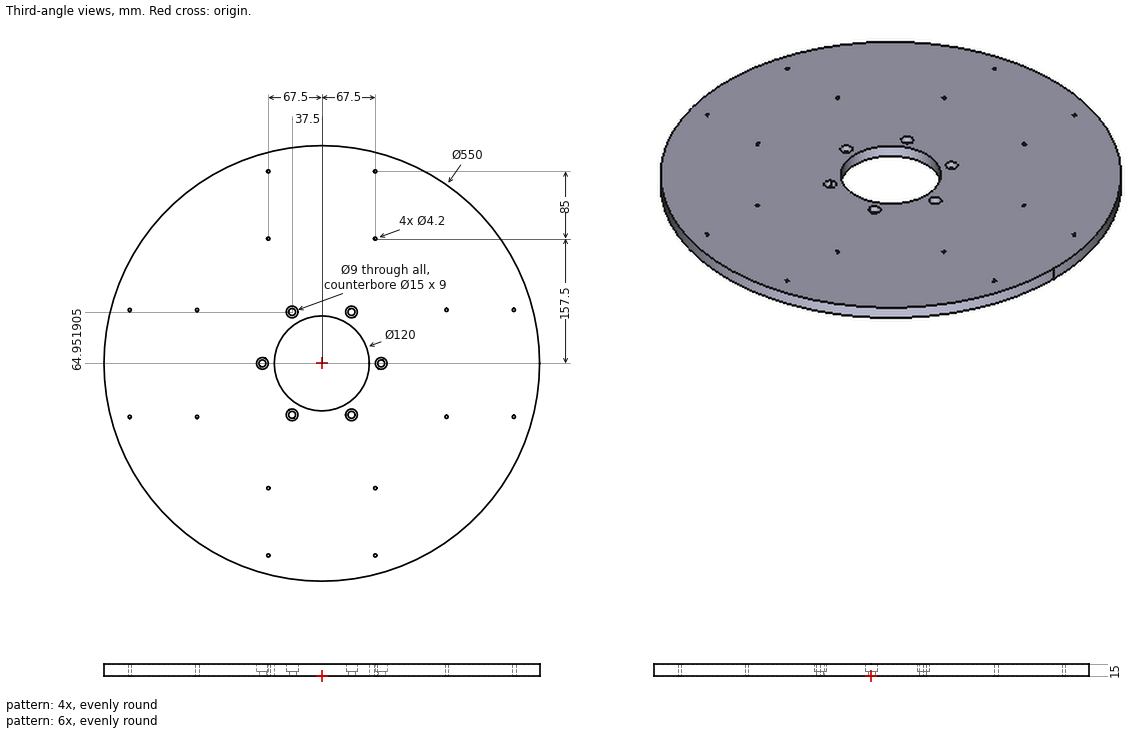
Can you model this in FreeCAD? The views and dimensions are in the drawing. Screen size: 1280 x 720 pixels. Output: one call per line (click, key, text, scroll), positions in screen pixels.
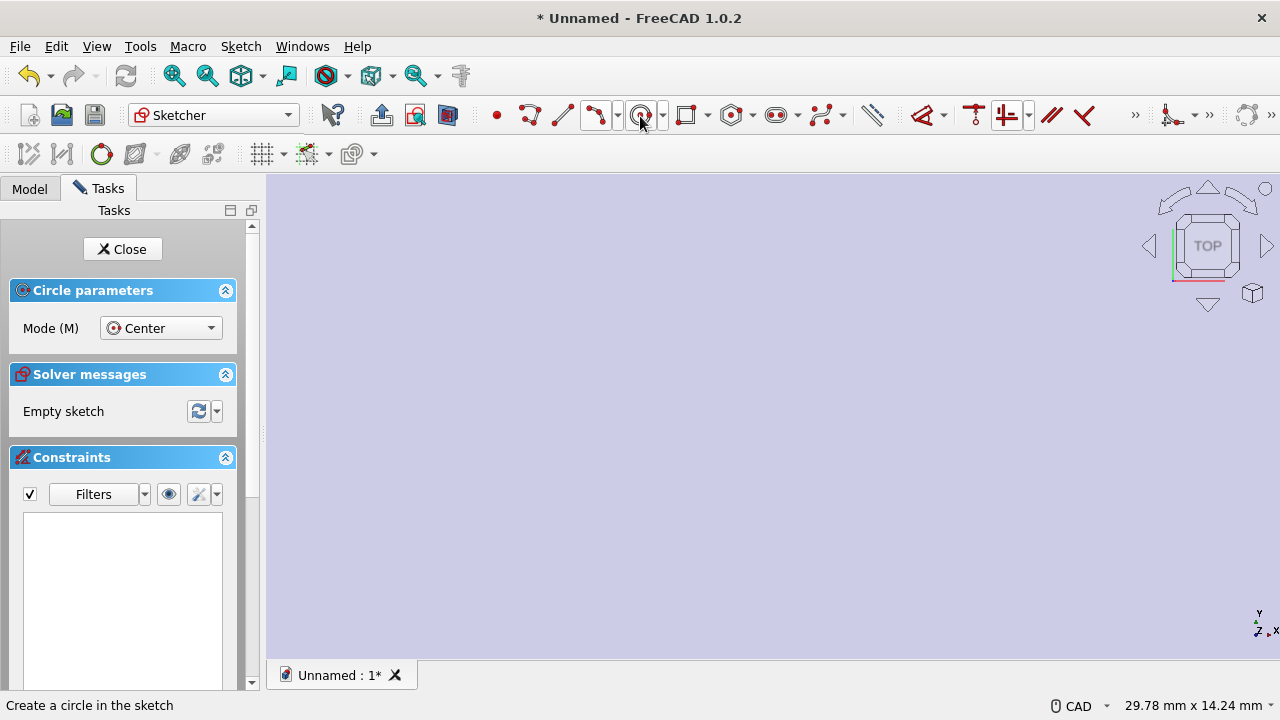
click(703, 416)
move(811, 307)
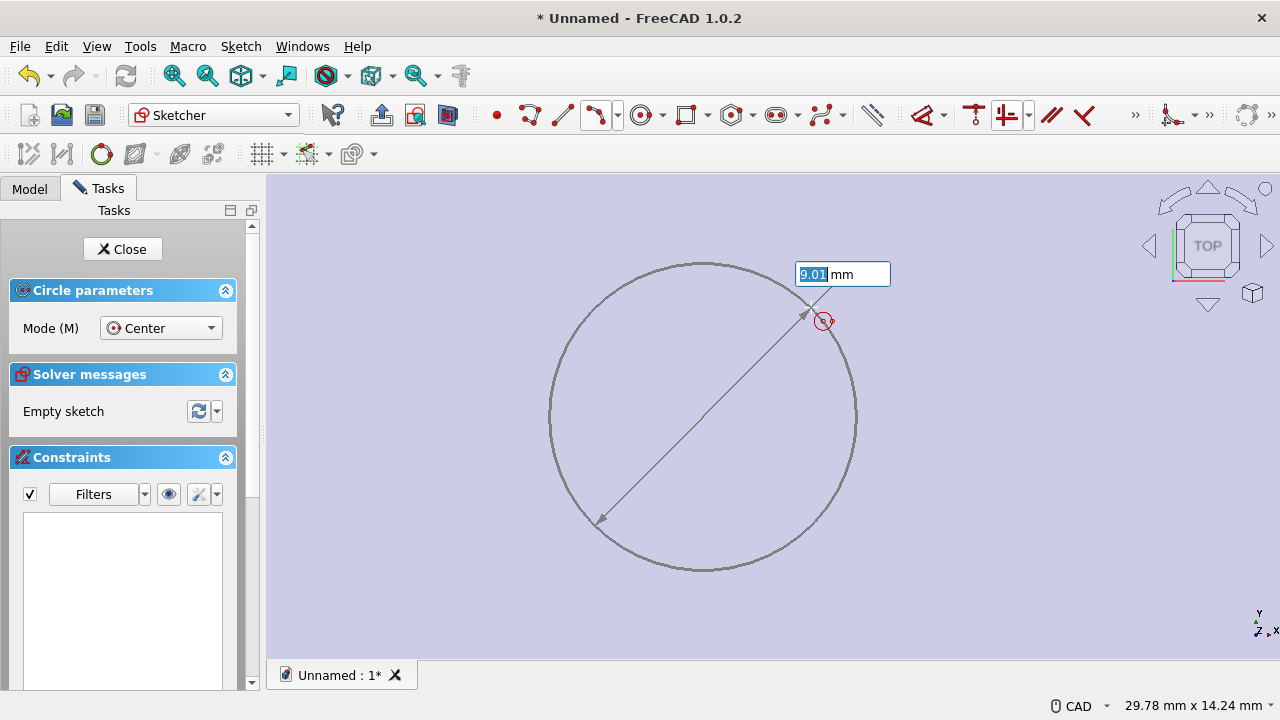
text(9)
key(Return)
key(Escape)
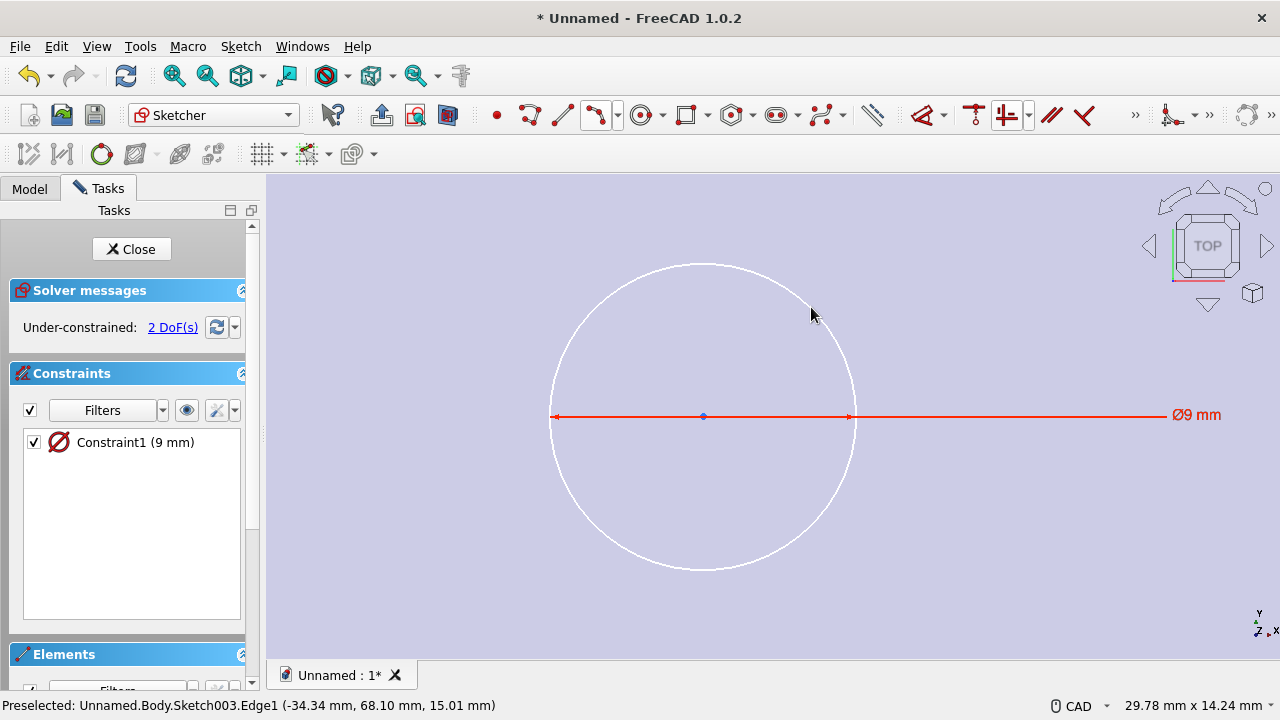
click(922, 116)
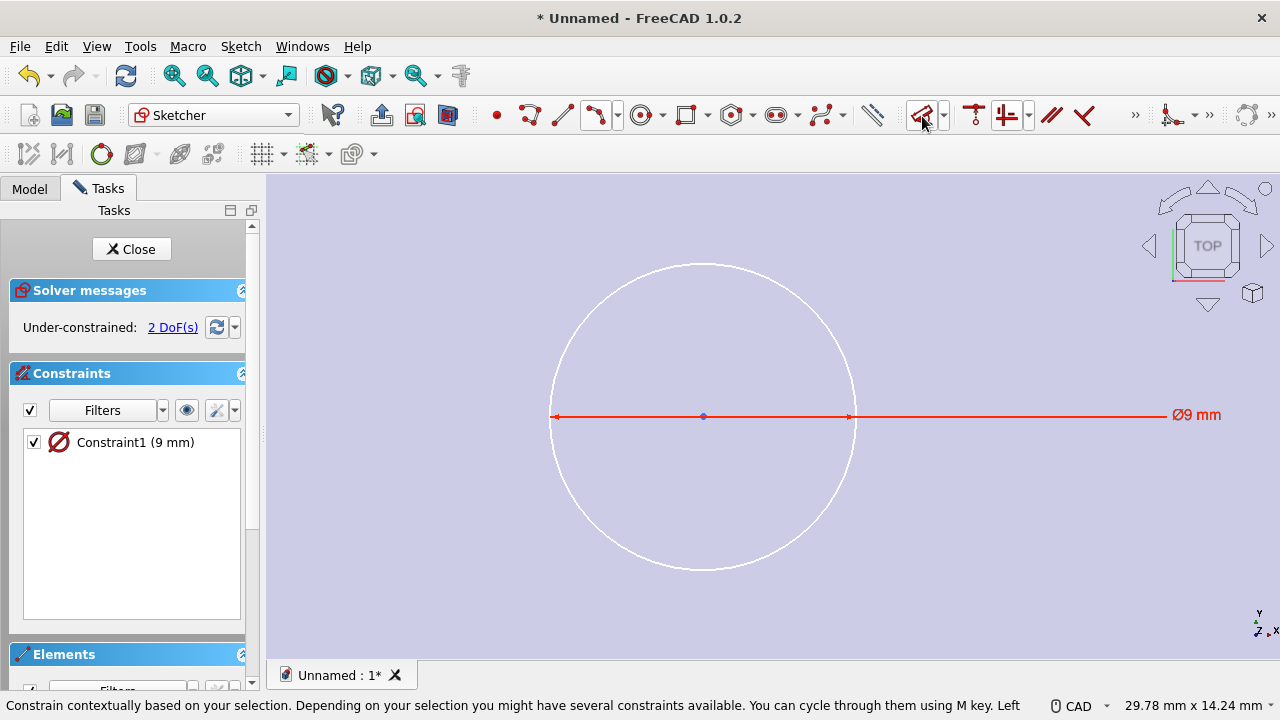
click(703, 417)
click(909, 383)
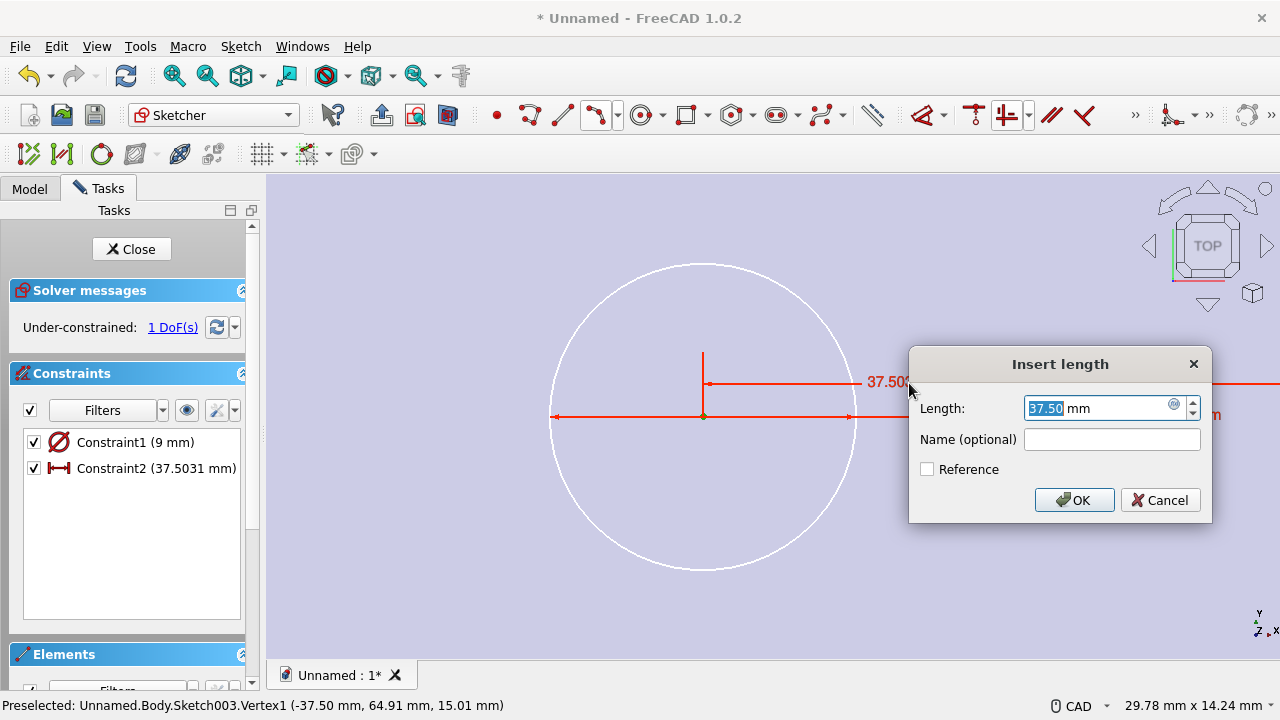
text(37.5)
key(Return)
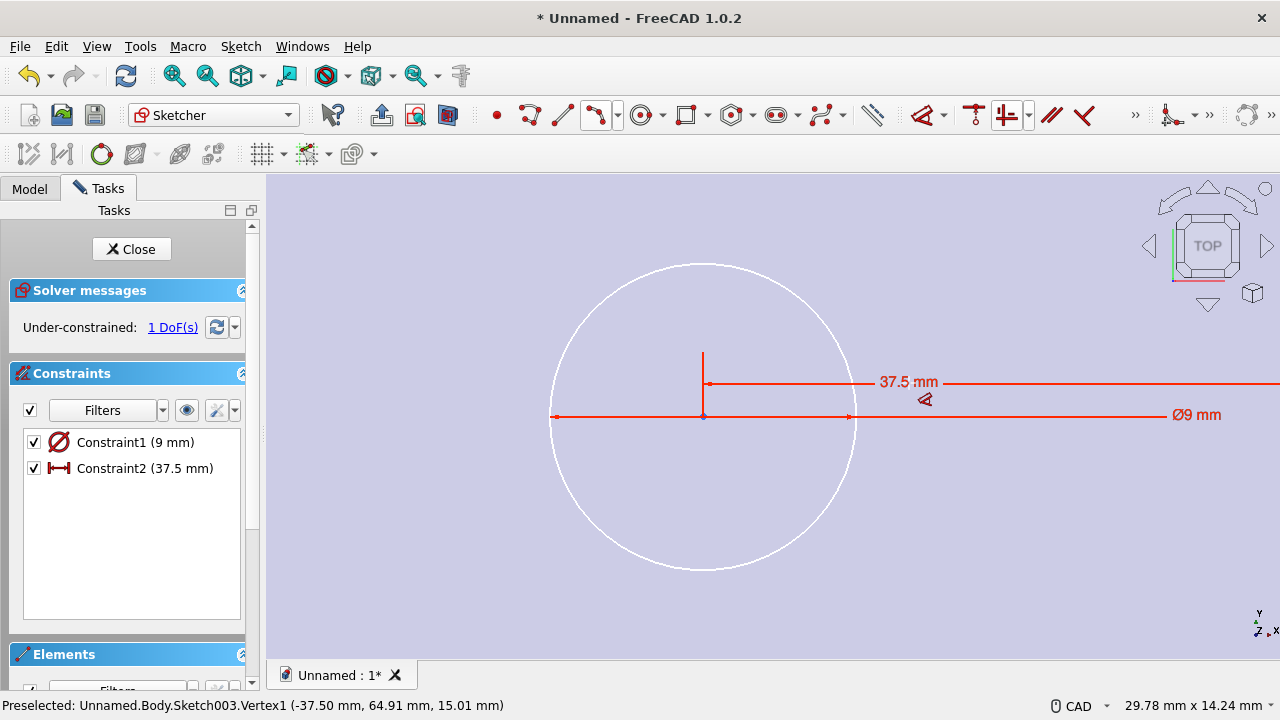
click(703, 417)
click(669, 524)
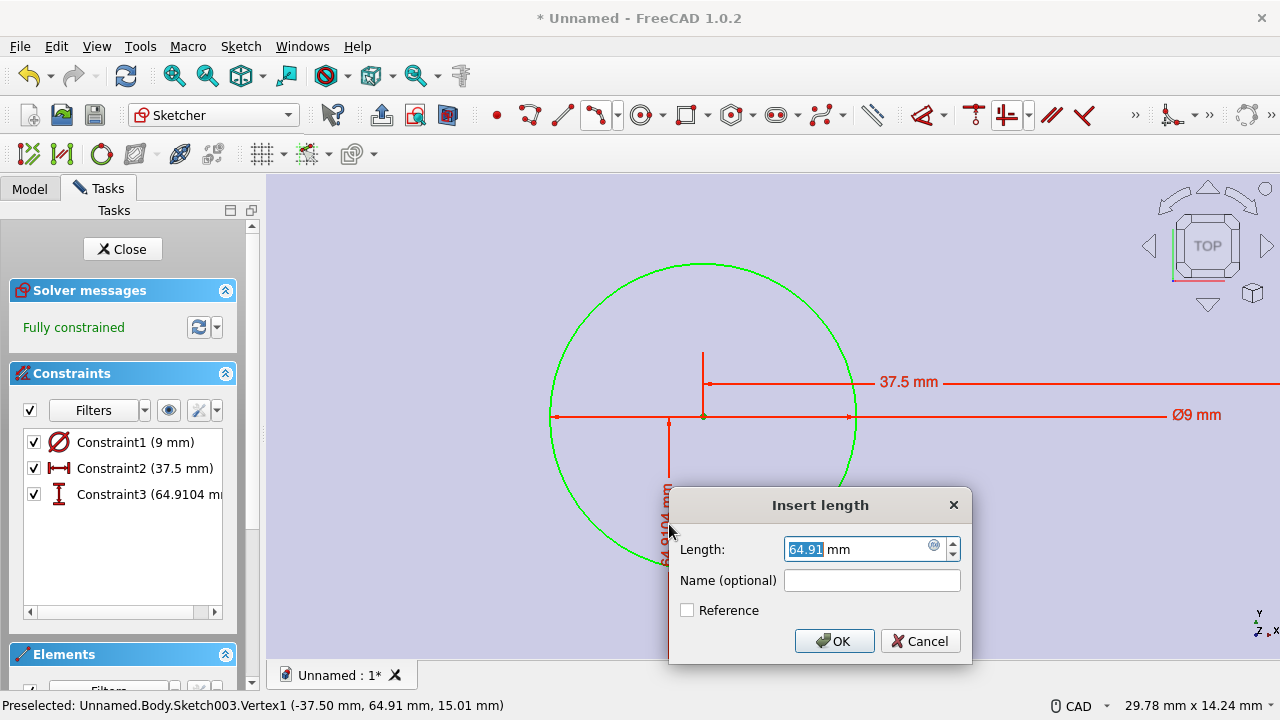
text(64.951905)
key(Return)
key(Escape)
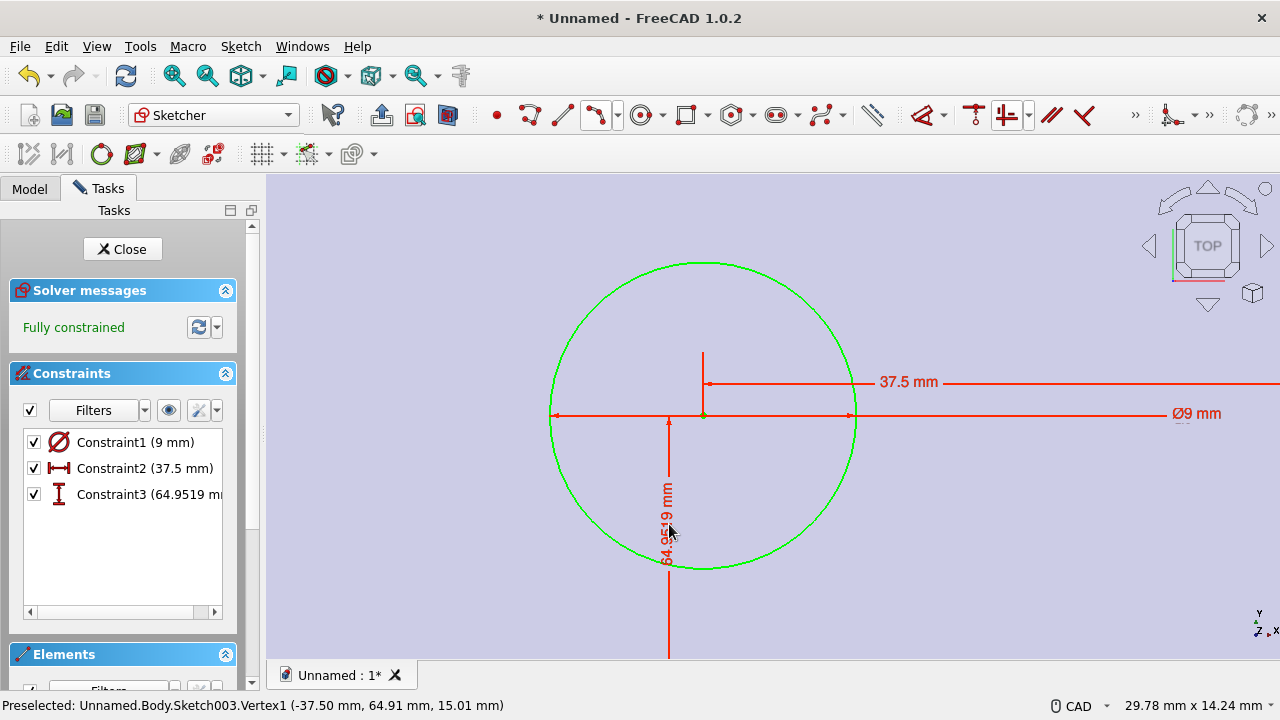
click(123, 249)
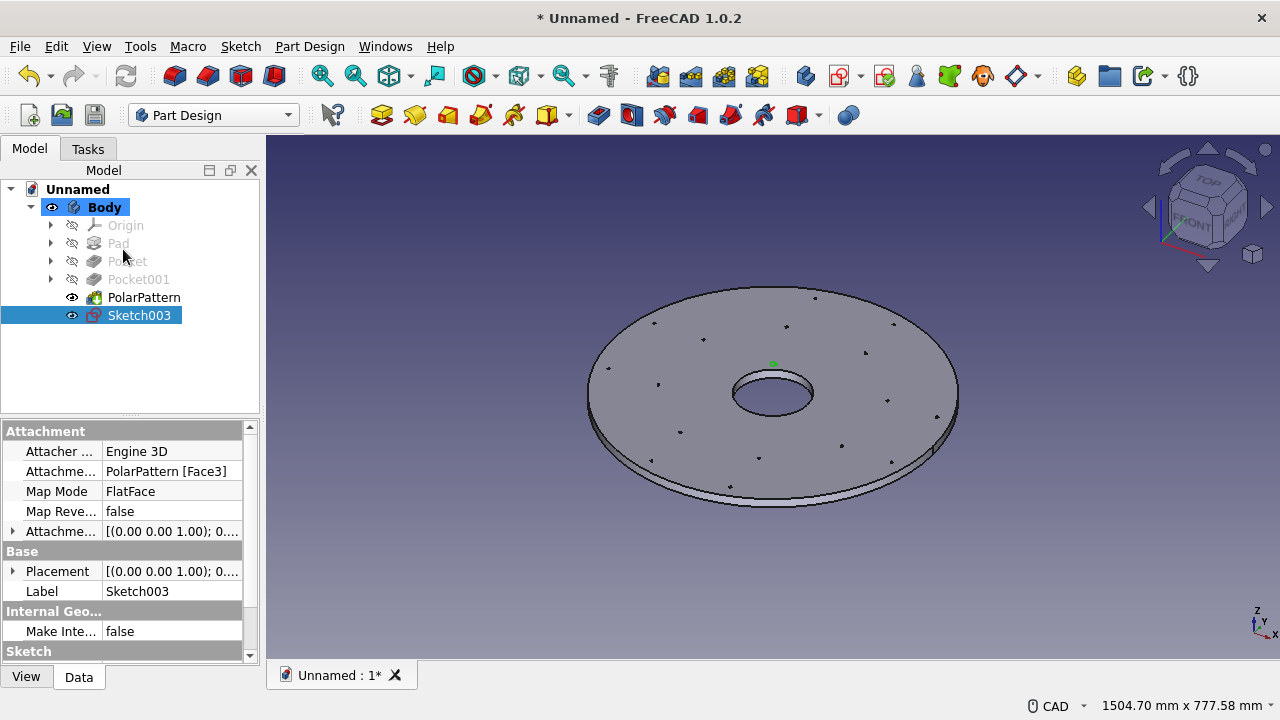
click(632, 116)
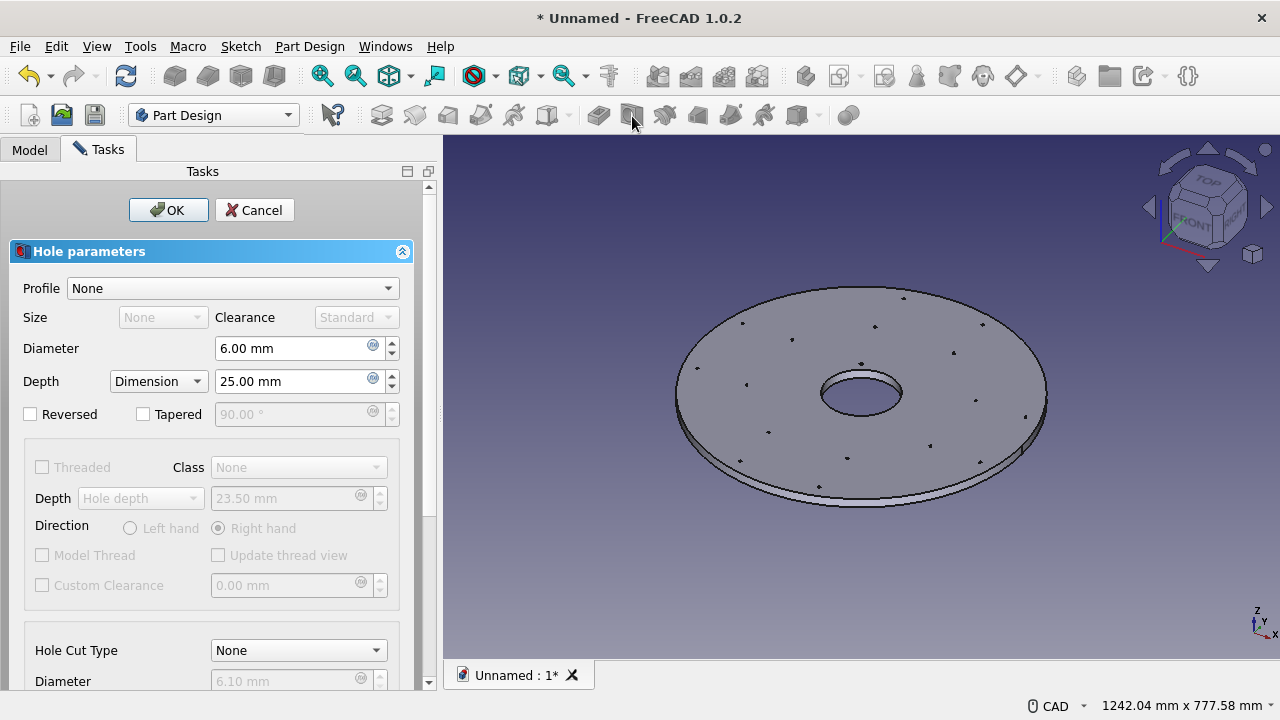
triple_click(300, 348)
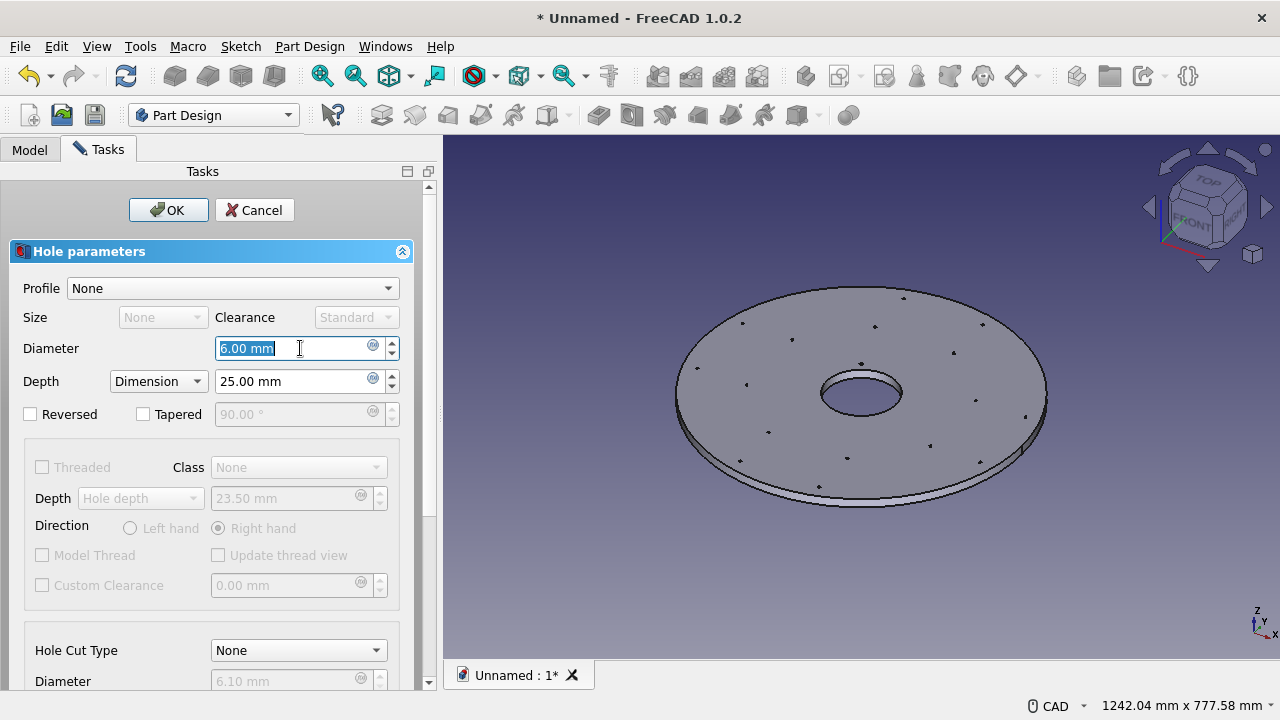
text(9)
key(Tab)